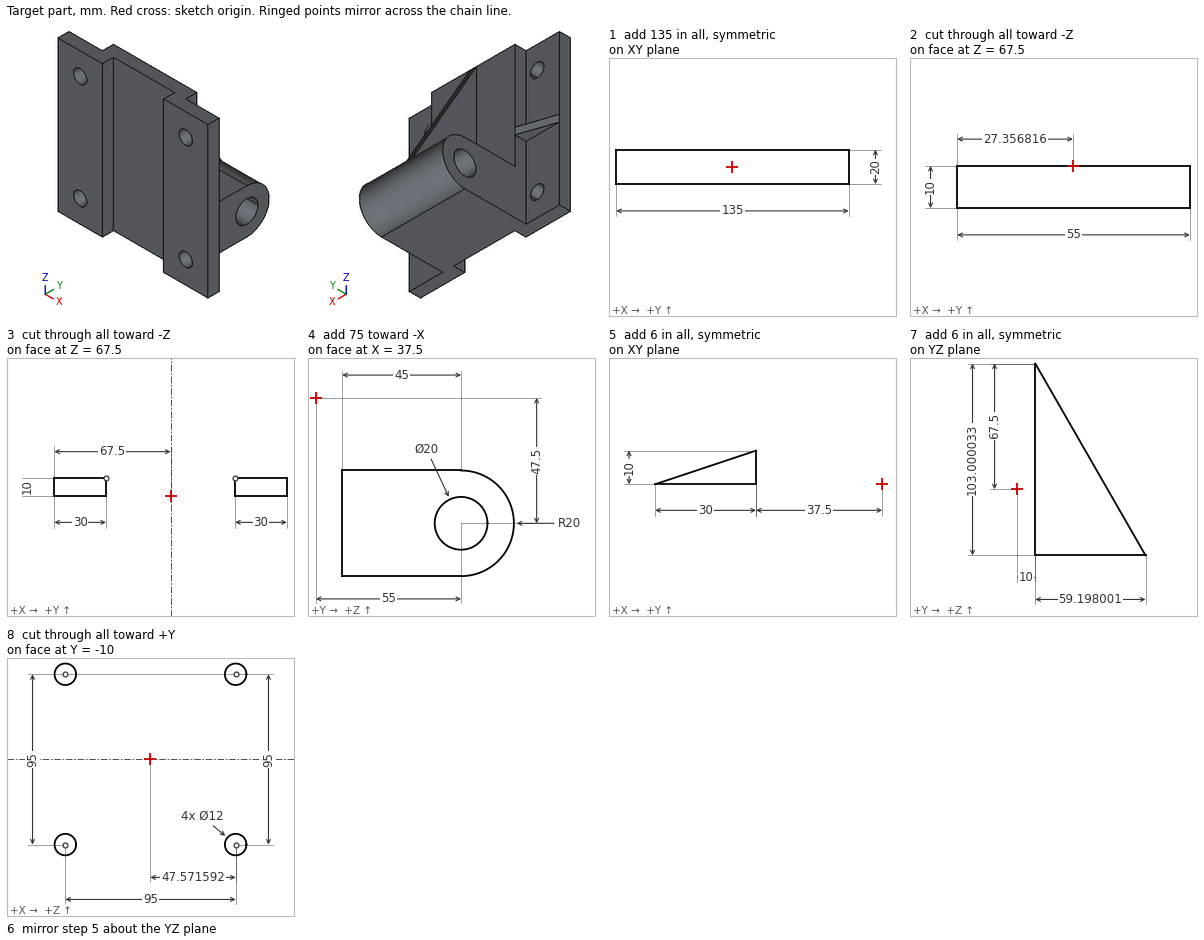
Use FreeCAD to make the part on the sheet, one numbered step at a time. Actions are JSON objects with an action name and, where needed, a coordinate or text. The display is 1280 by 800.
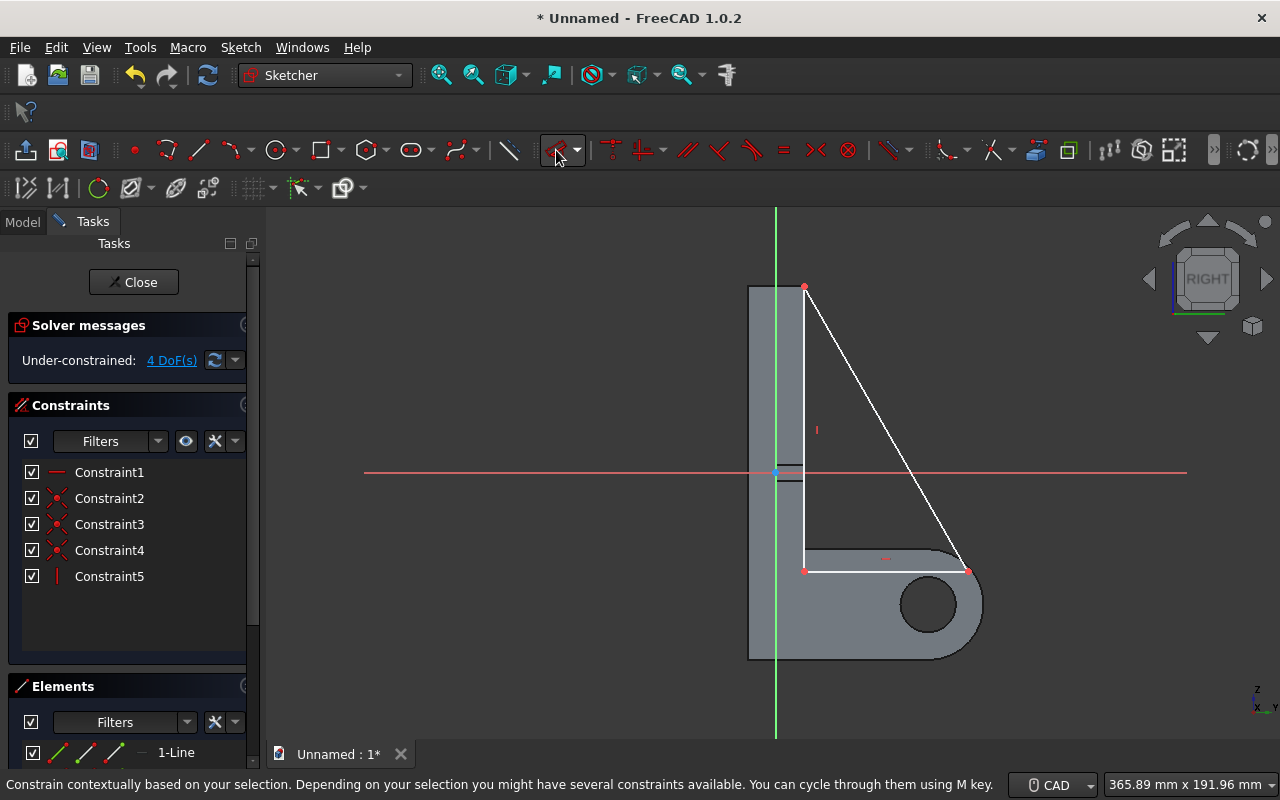
{"action": "scroll", "coordinate": [804, 572], "scroll_direction": "up", "scroll_amount": 2}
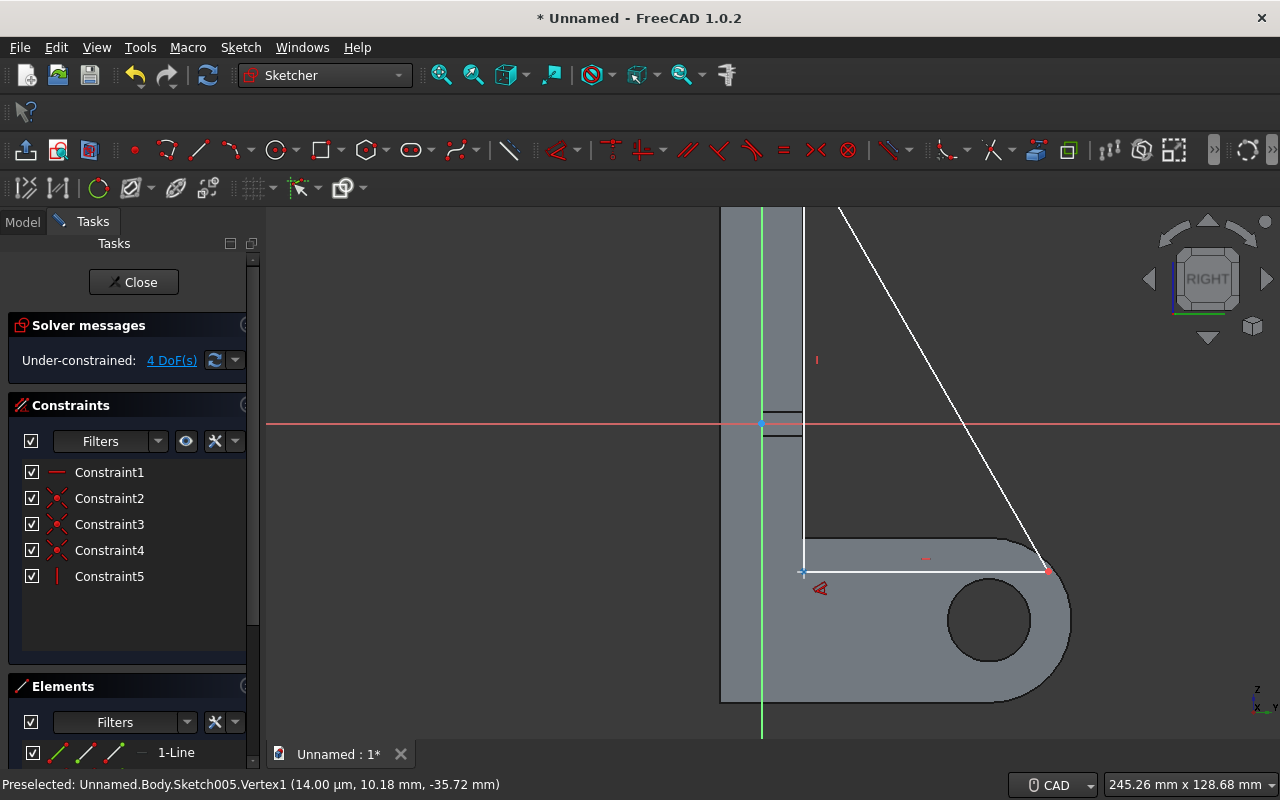
{"action": "left_click", "coordinate": [804, 572]}
{"action": "left_click", "coordinate": [783, 606]}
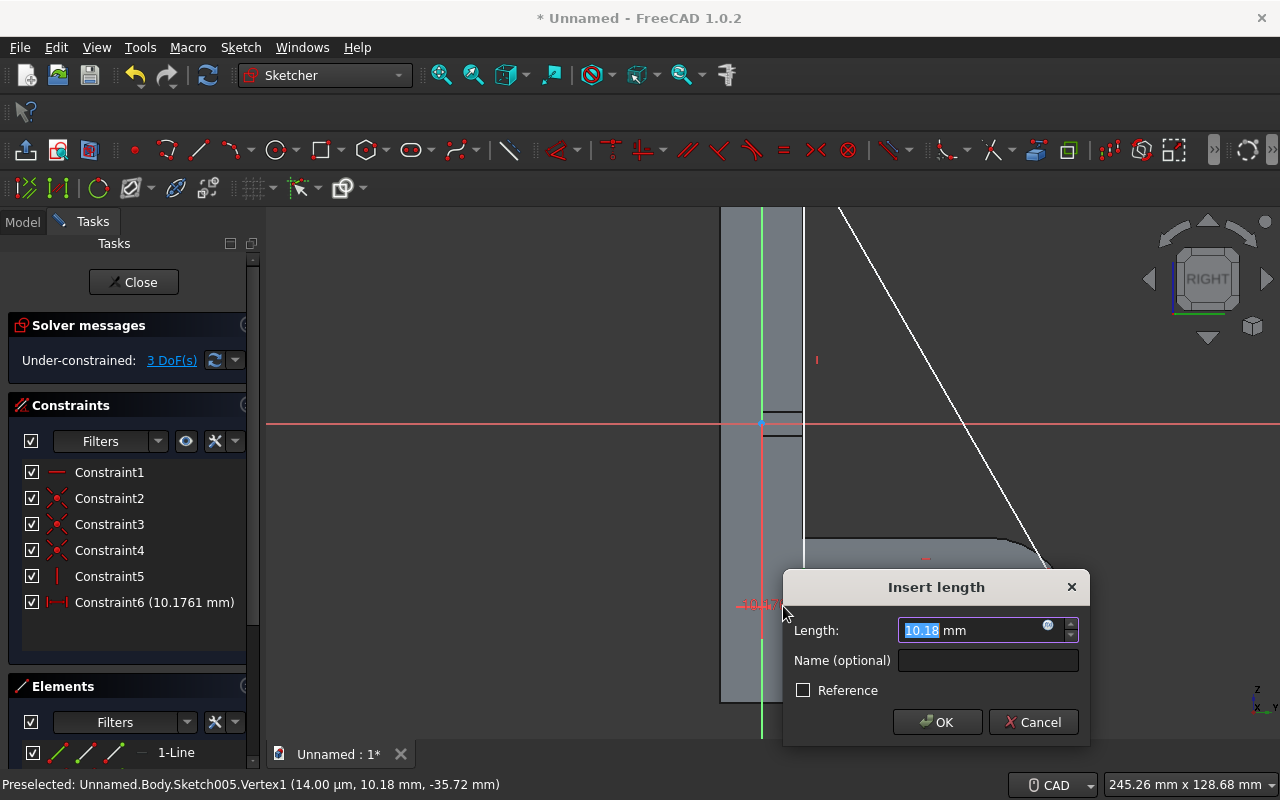
{"action": "type", "text": "10"}
{"action": "key", "text": "Return"}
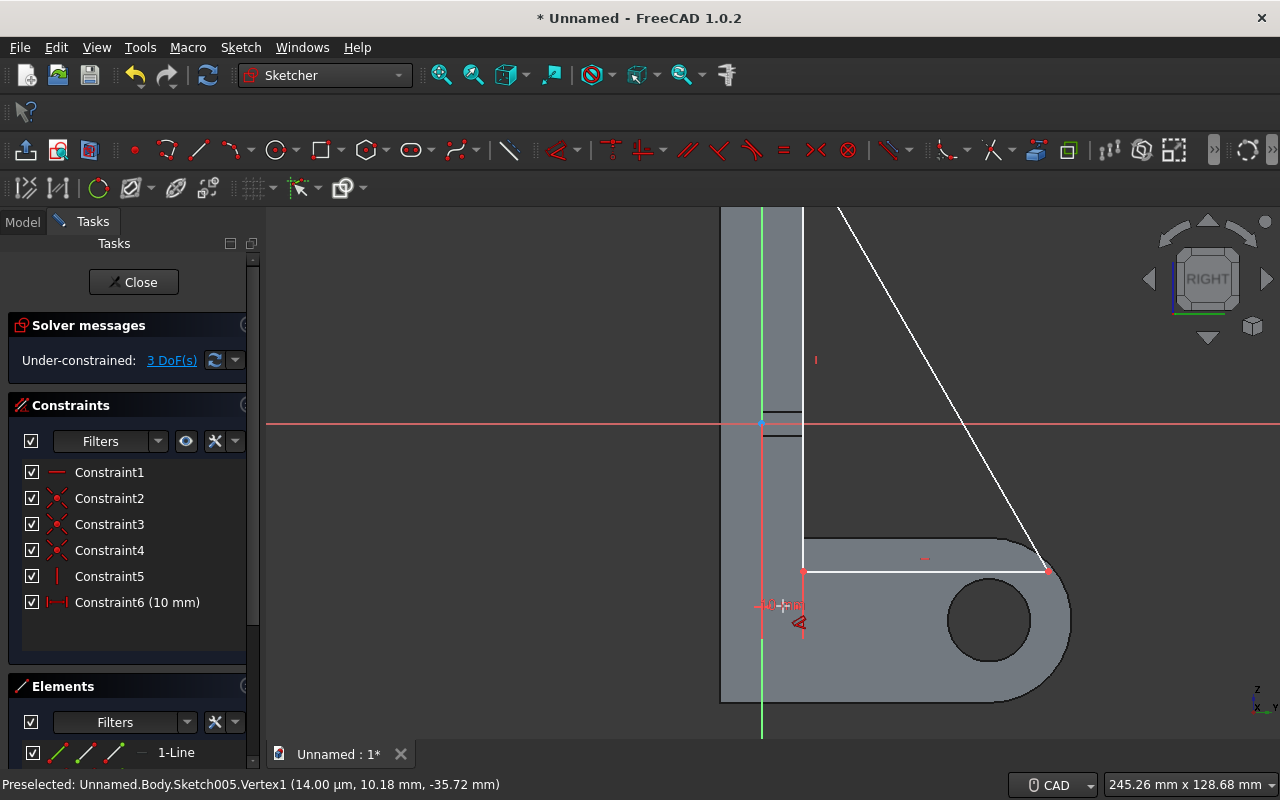
{"action": "scroll", "coordinate": [297, 707], "scroll_direction": "down", "scroll_amount": 2}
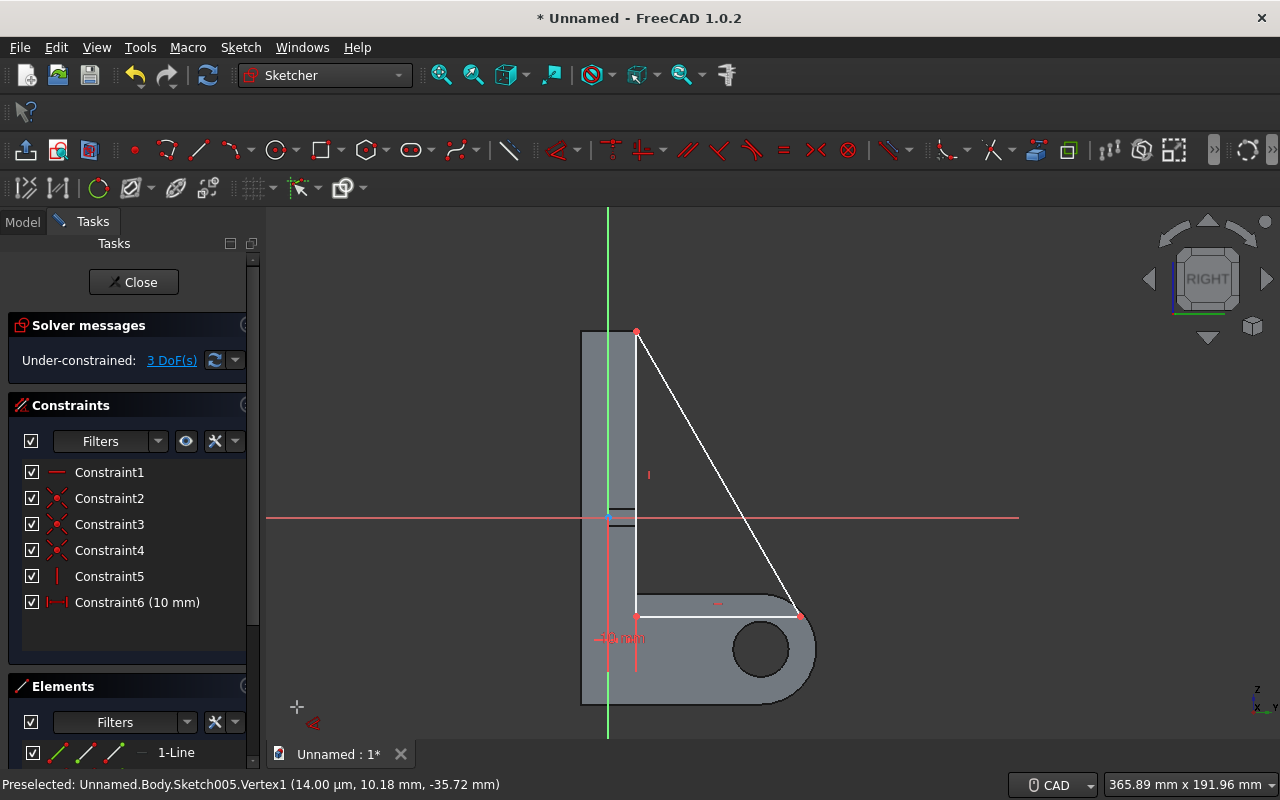
{"action": "left_click", "coordinate": [636, 332]}
{"action": "left_click", "coordinate": [574, 425]}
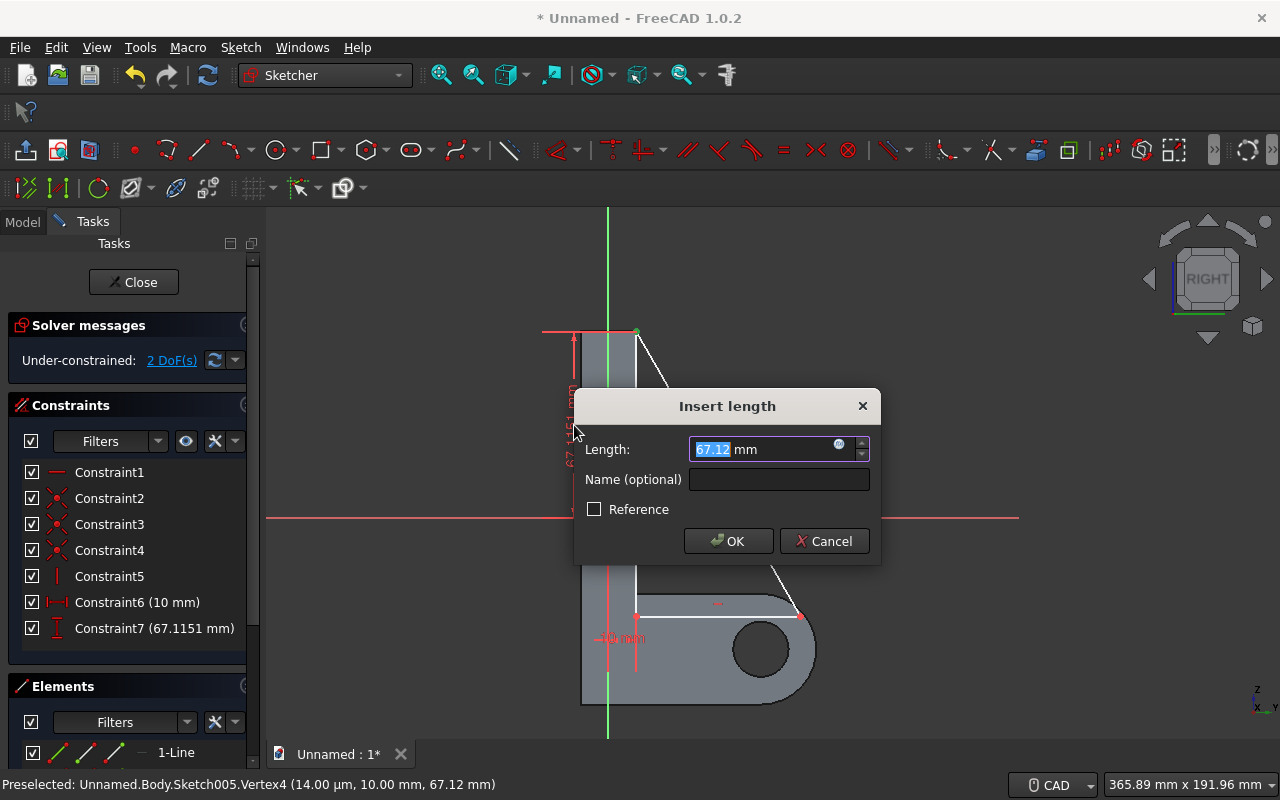
{"action": "type", "text": "67.5"}
{"action": "key", "text": "Return"}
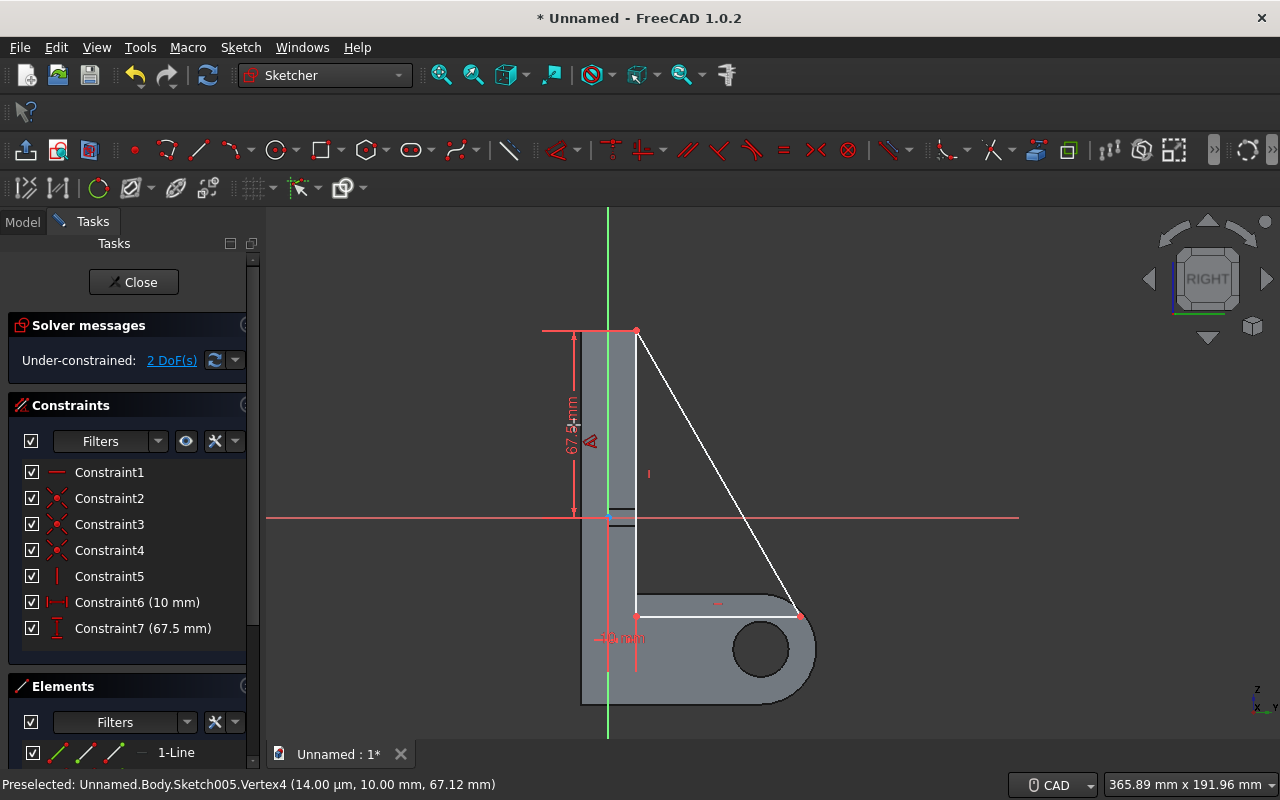
{"action": "left_click", "coordinate": [686, 617]}
{"action": "left_click", "coordinate": [718, 651]}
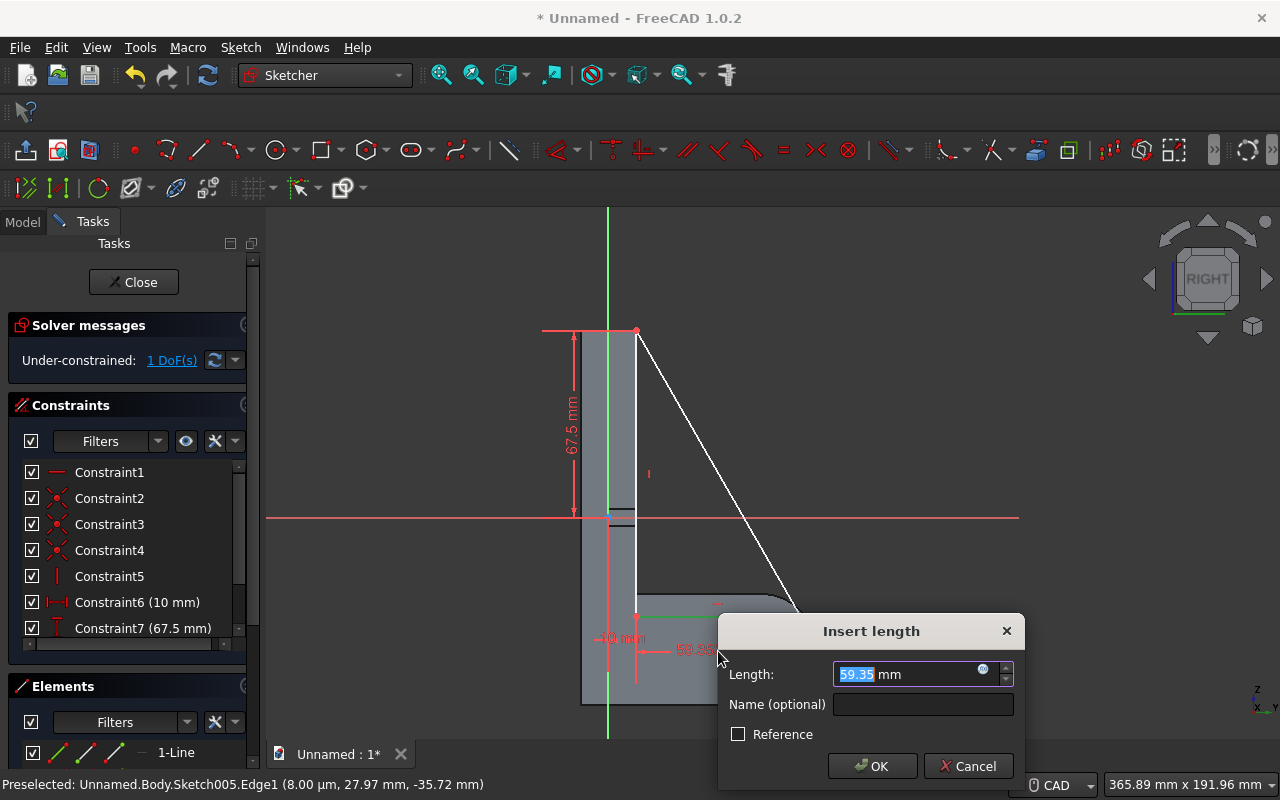
{"action": "type", "text": "59.198001"}
{"action": "key", "text": "Return"}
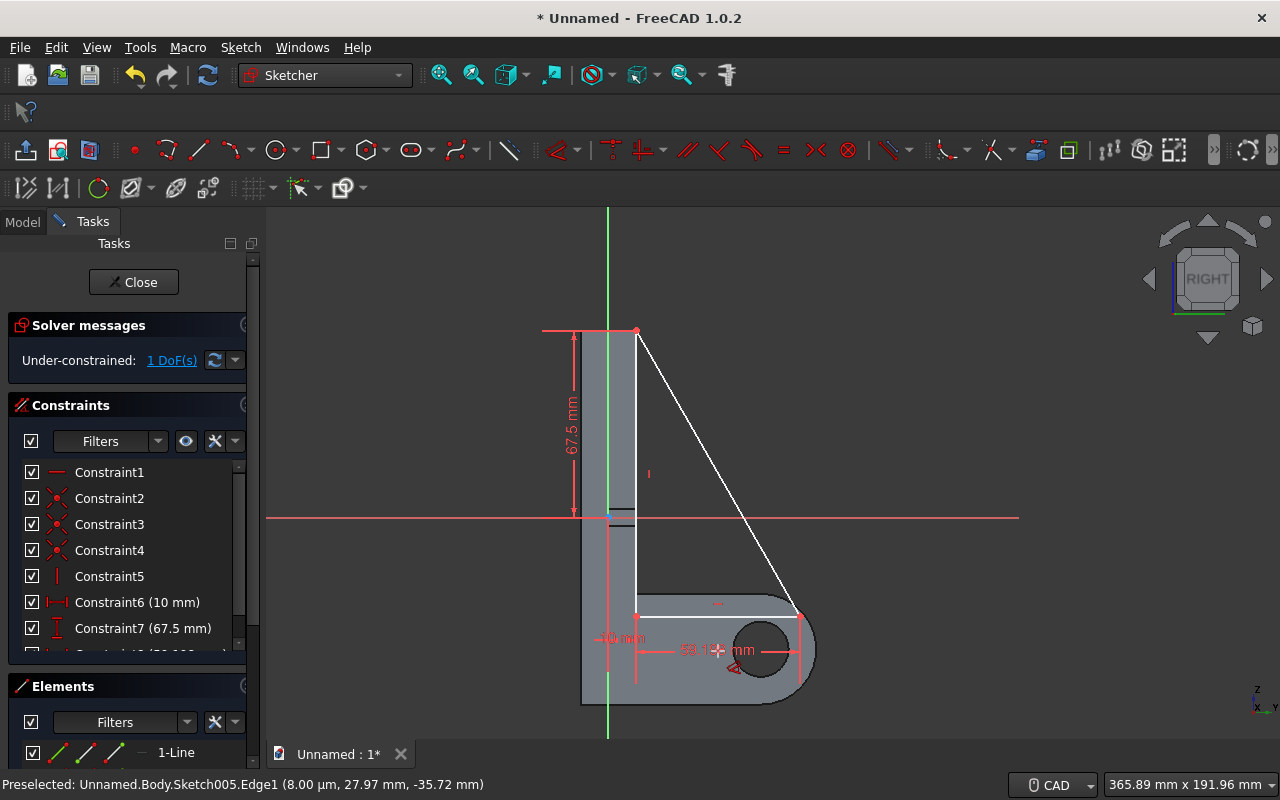
{"action": "left_click", "coordinate": [636, 416]}
{"action": "left_click", "coordinate": [670, 474]}